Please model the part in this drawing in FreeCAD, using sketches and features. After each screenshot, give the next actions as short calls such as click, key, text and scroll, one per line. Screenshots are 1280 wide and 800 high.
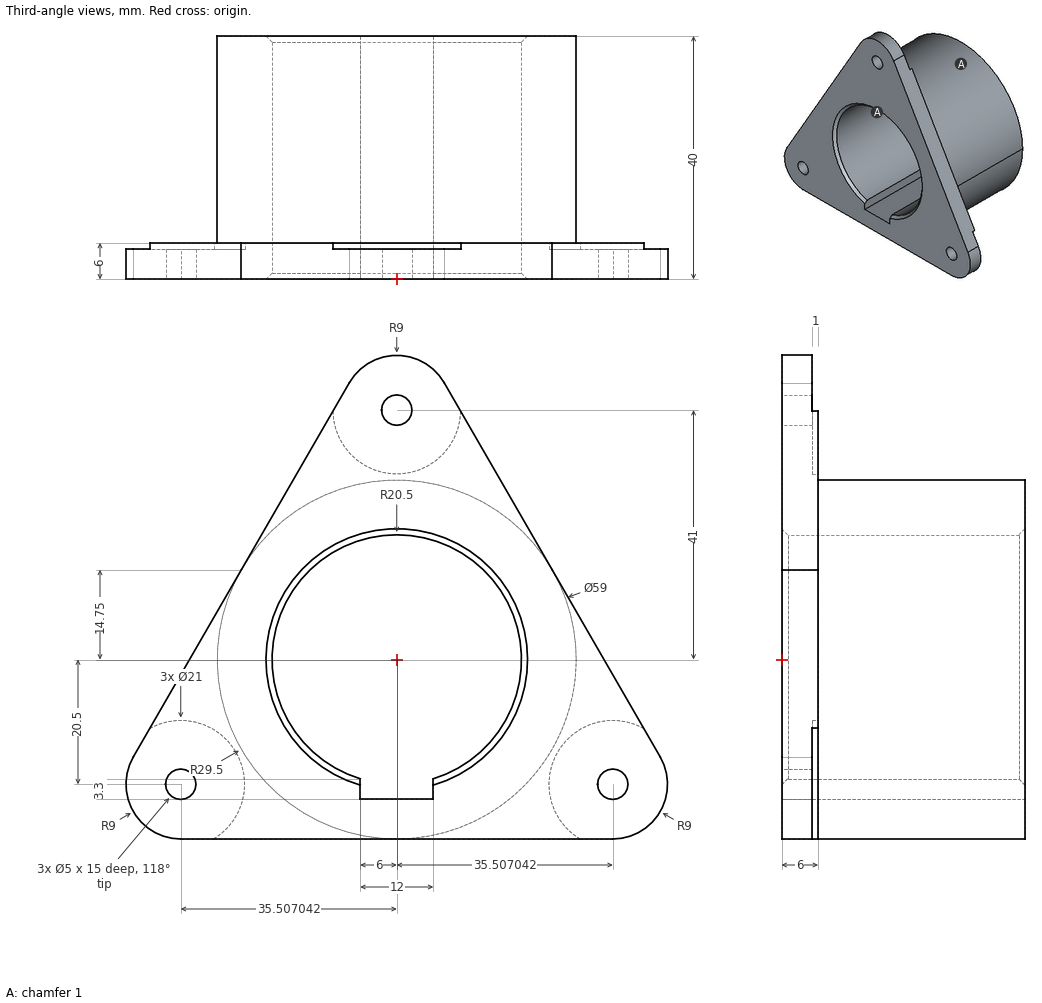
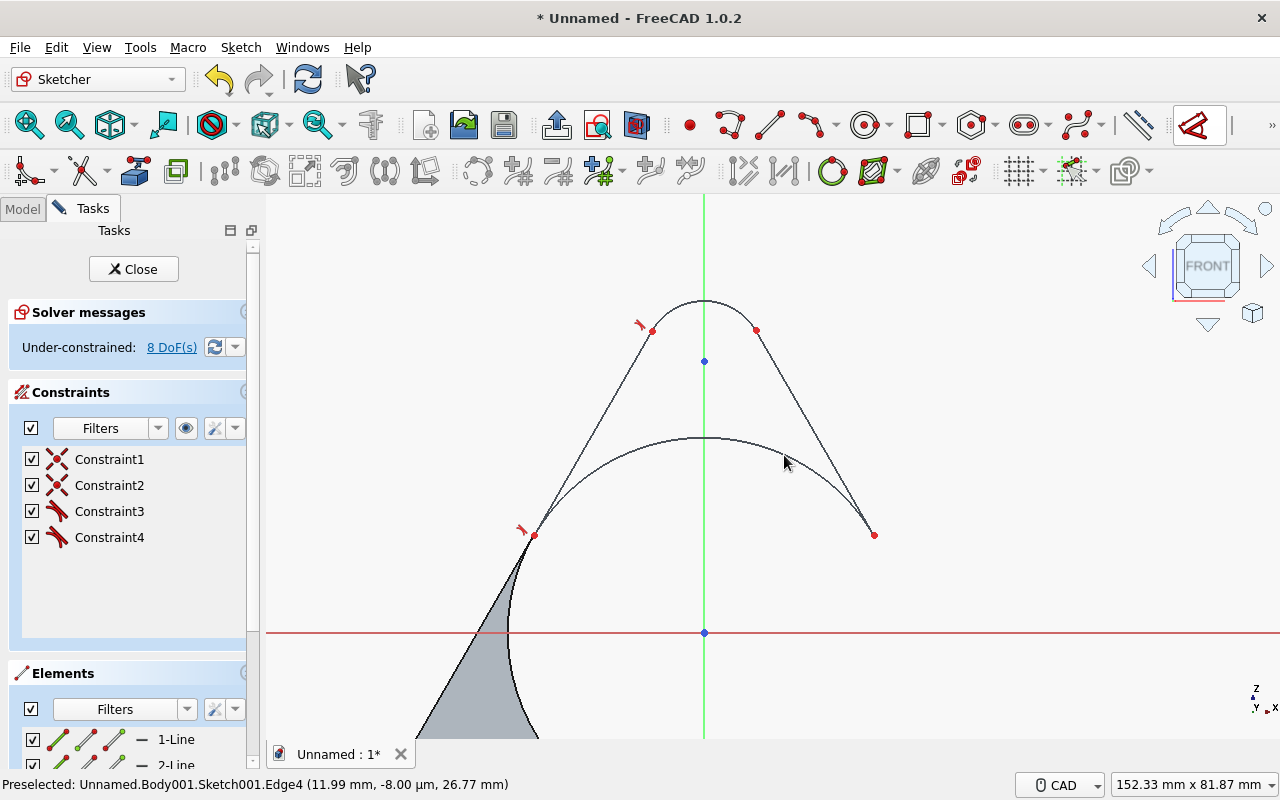
click(791, 393)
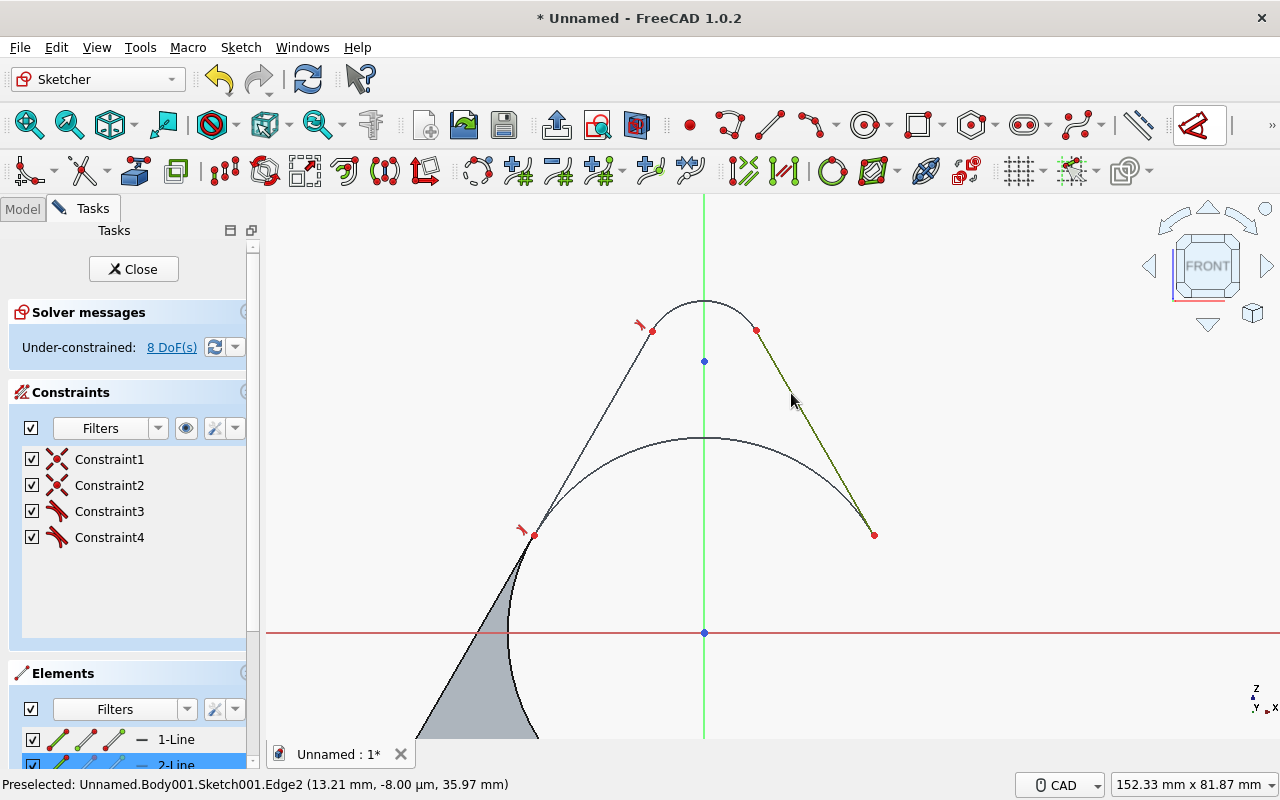
click(728, 306)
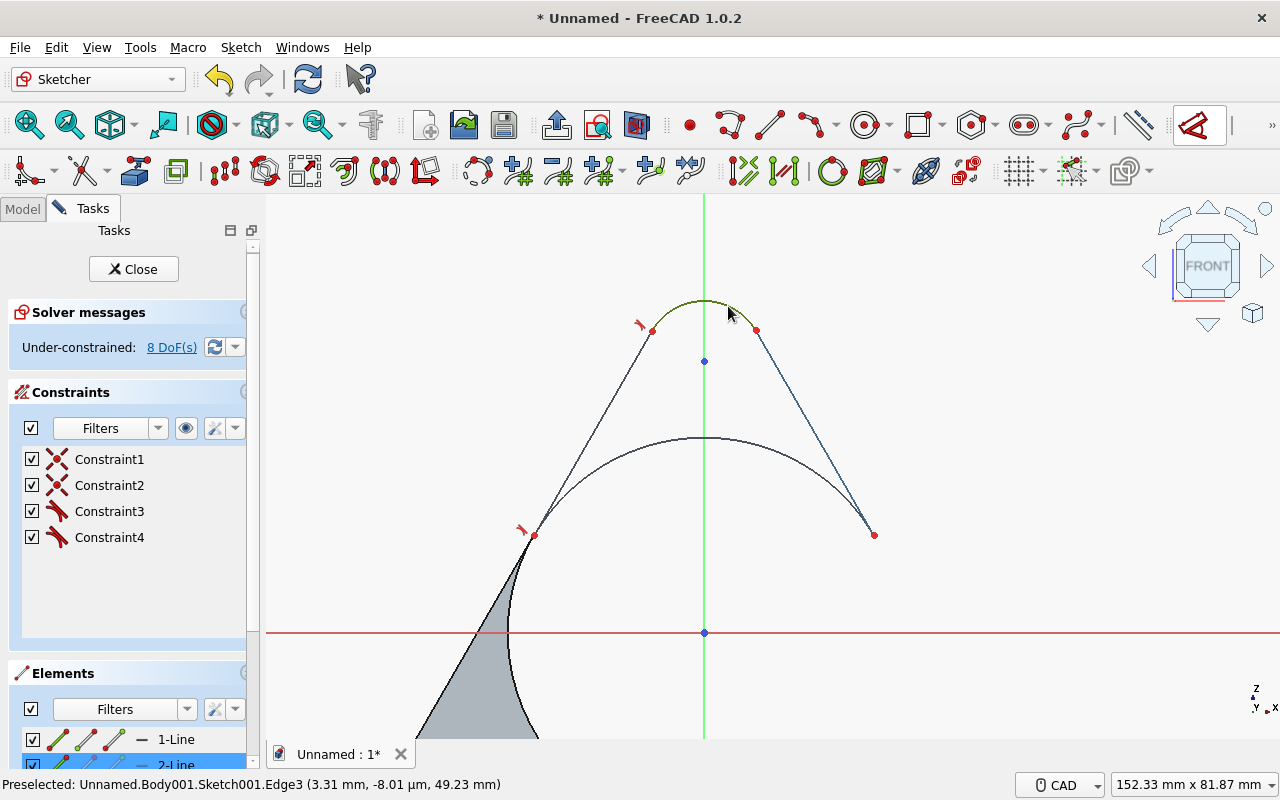
key(t)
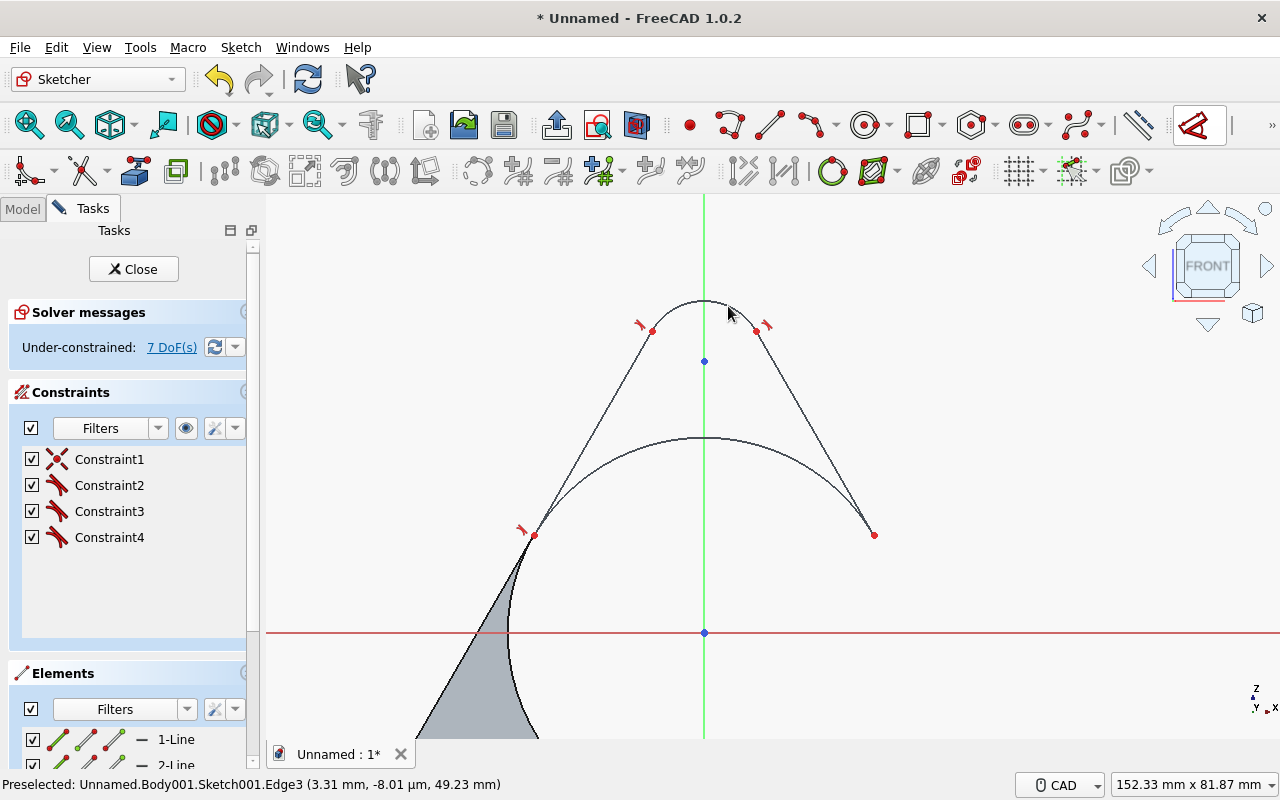
click(791, 393)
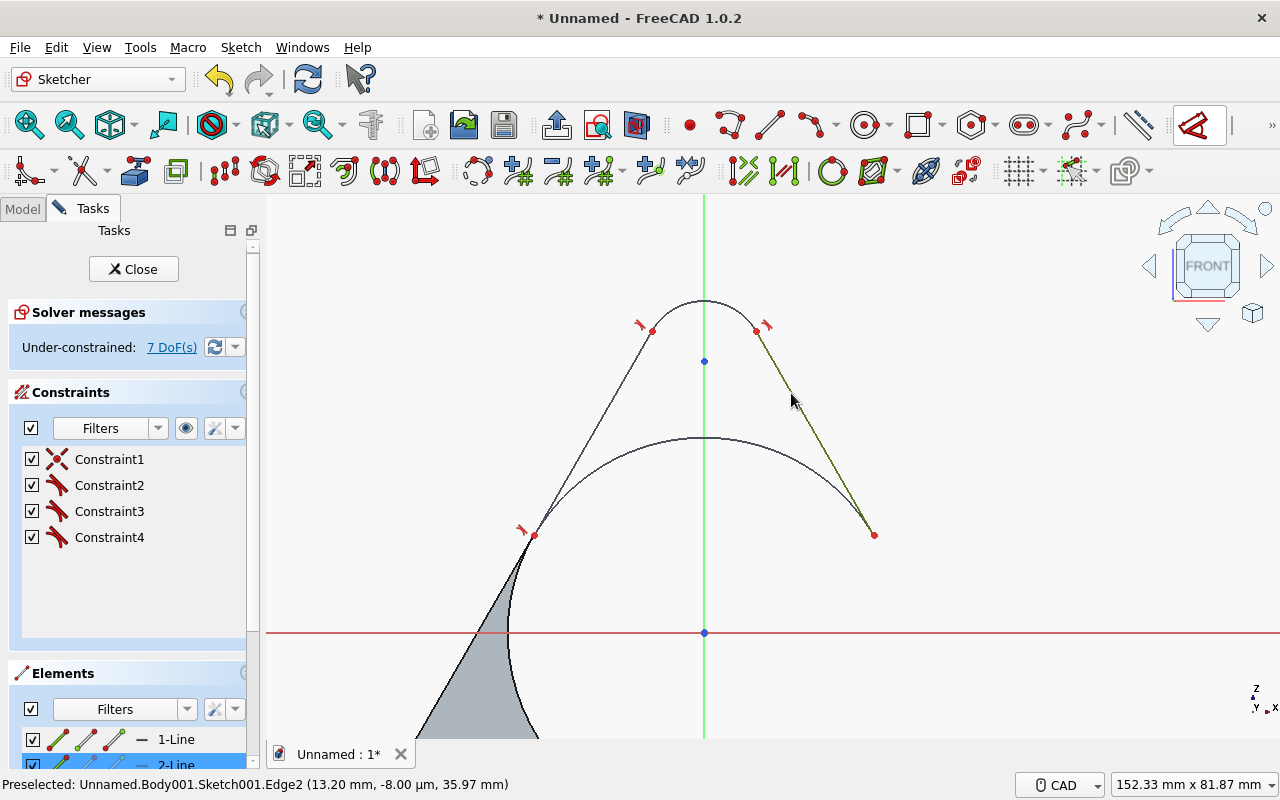
click(784, 455)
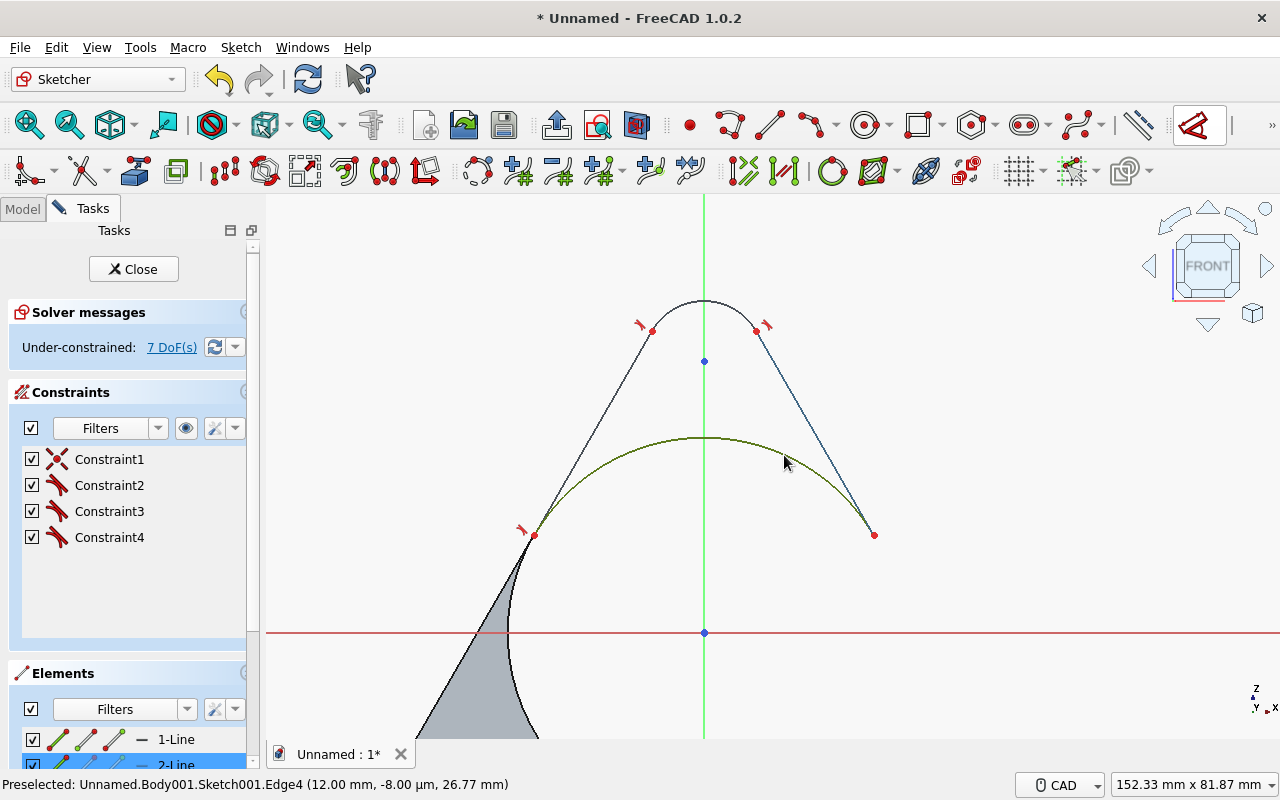
key(t)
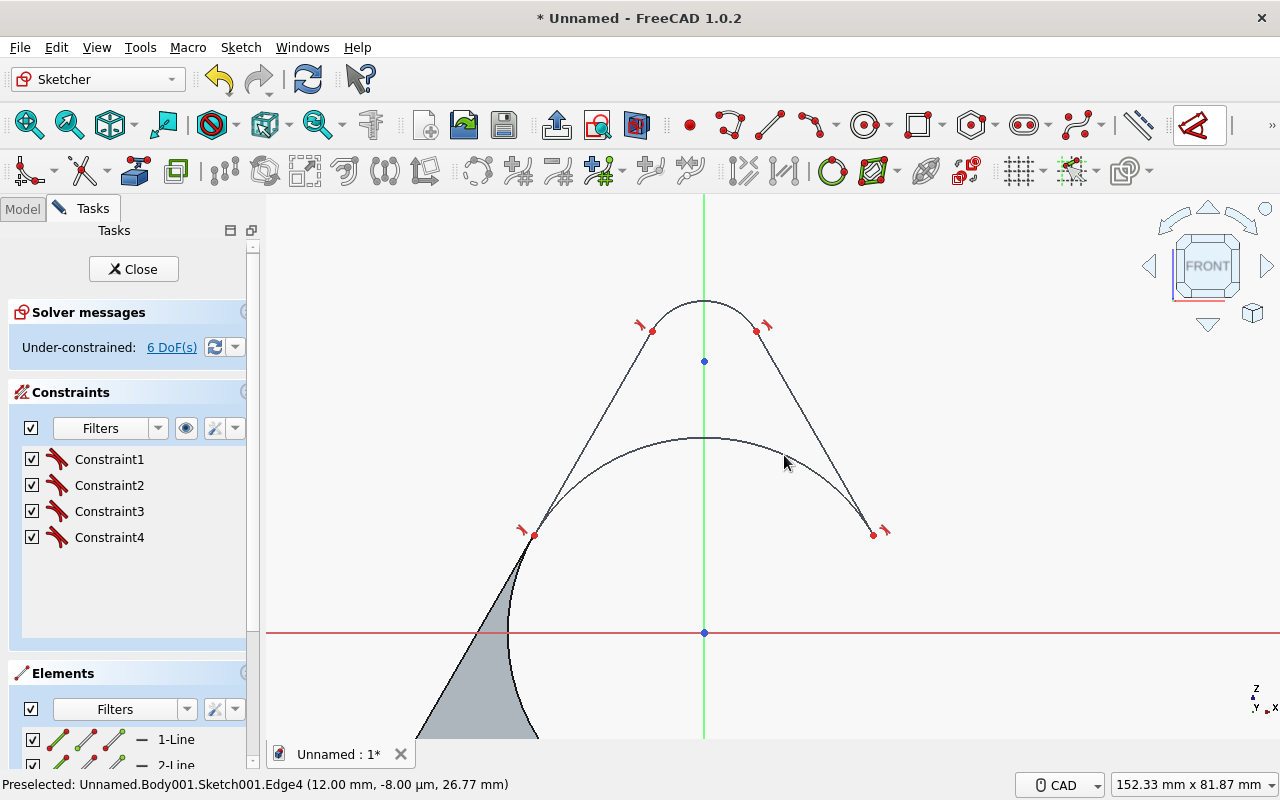
drag(694, 623, 714, 644)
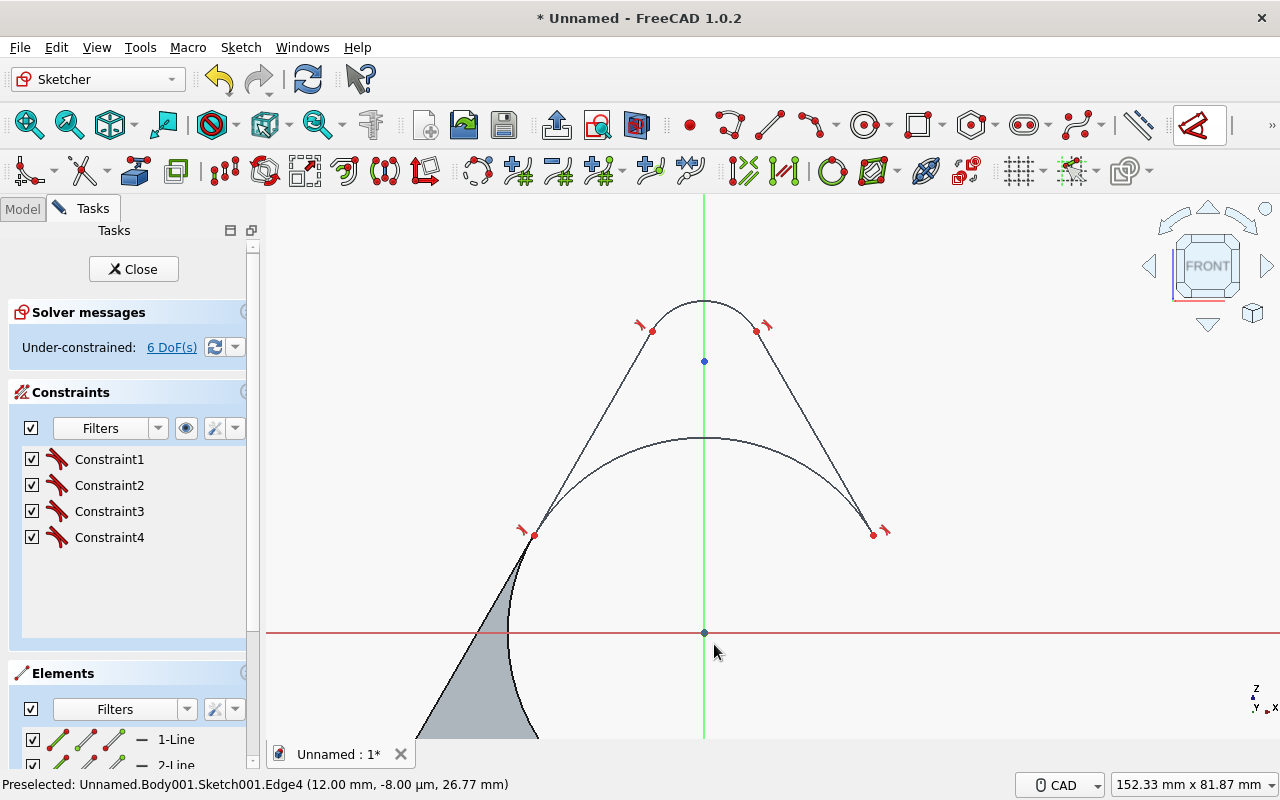
key(c)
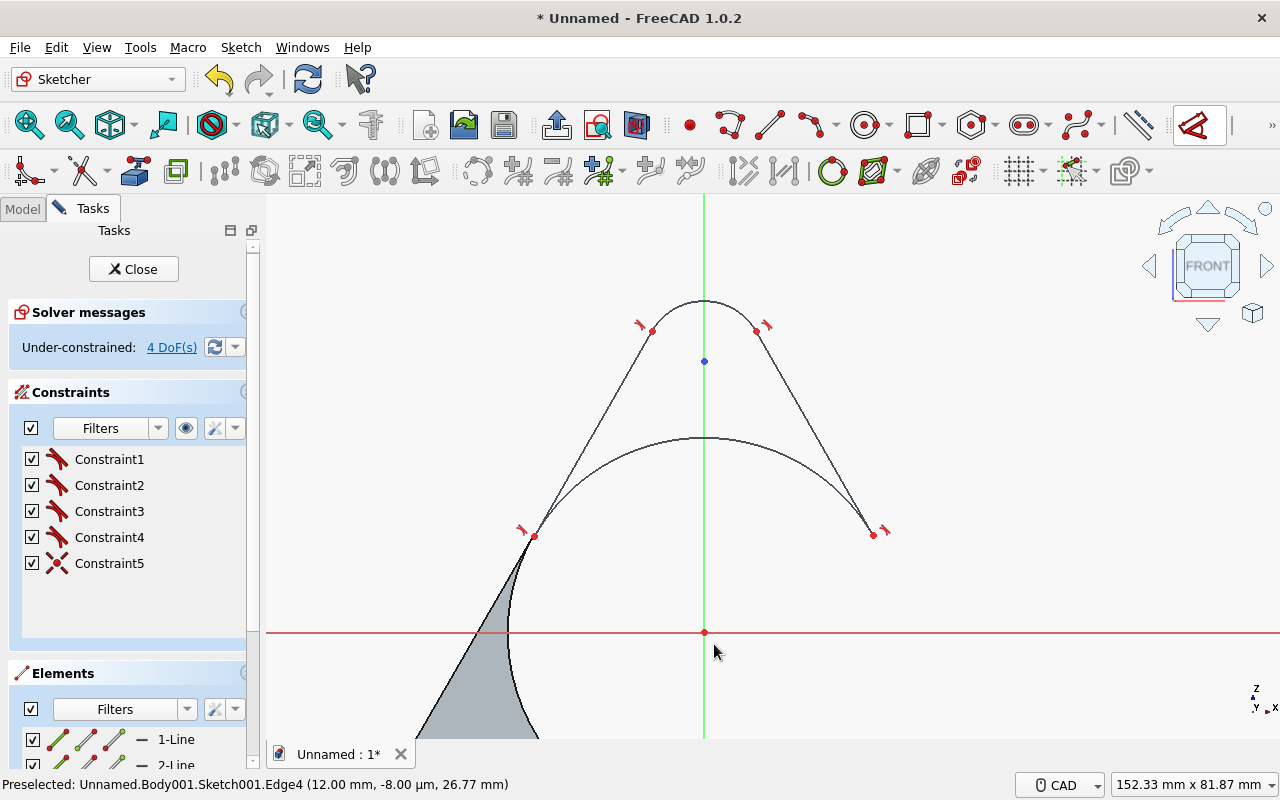
click(704, 361)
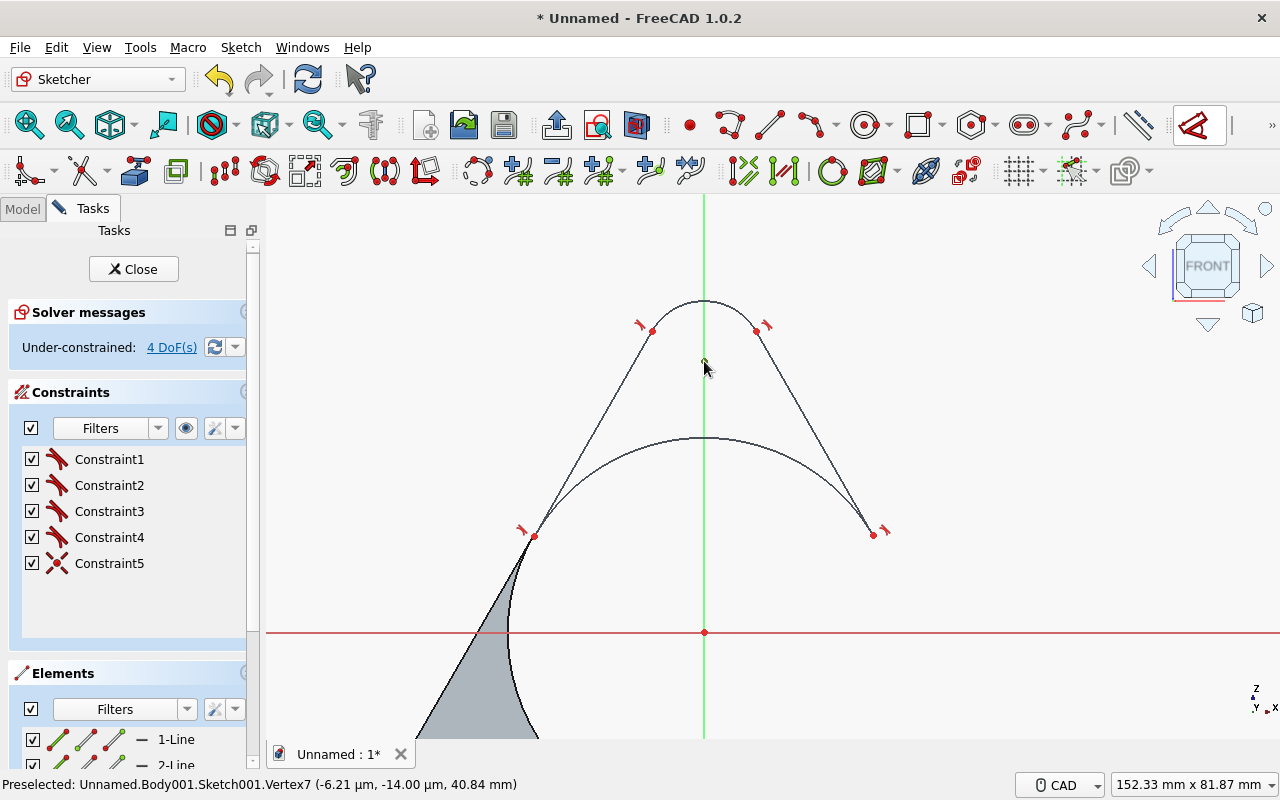
click(704, 676)